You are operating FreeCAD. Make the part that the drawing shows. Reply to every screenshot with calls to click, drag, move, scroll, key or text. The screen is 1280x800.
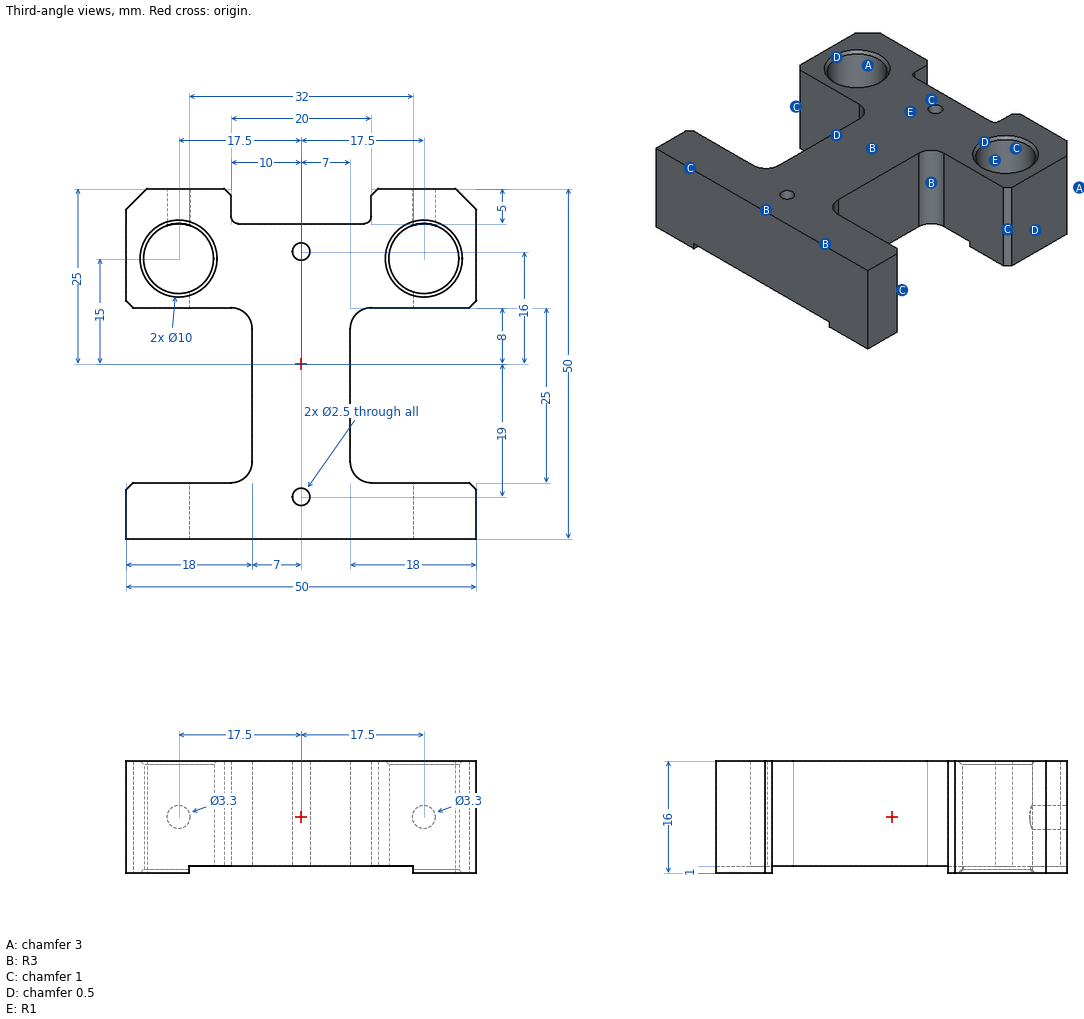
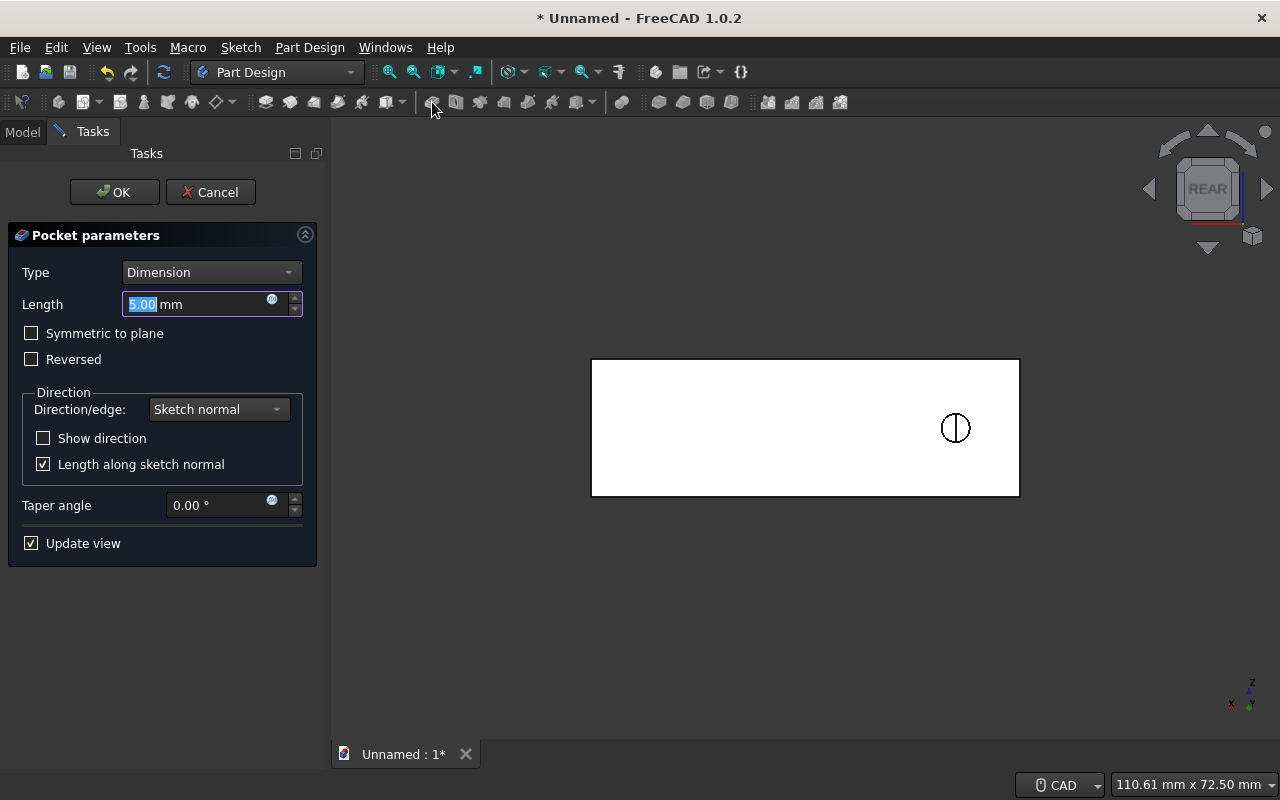
click(212, 272)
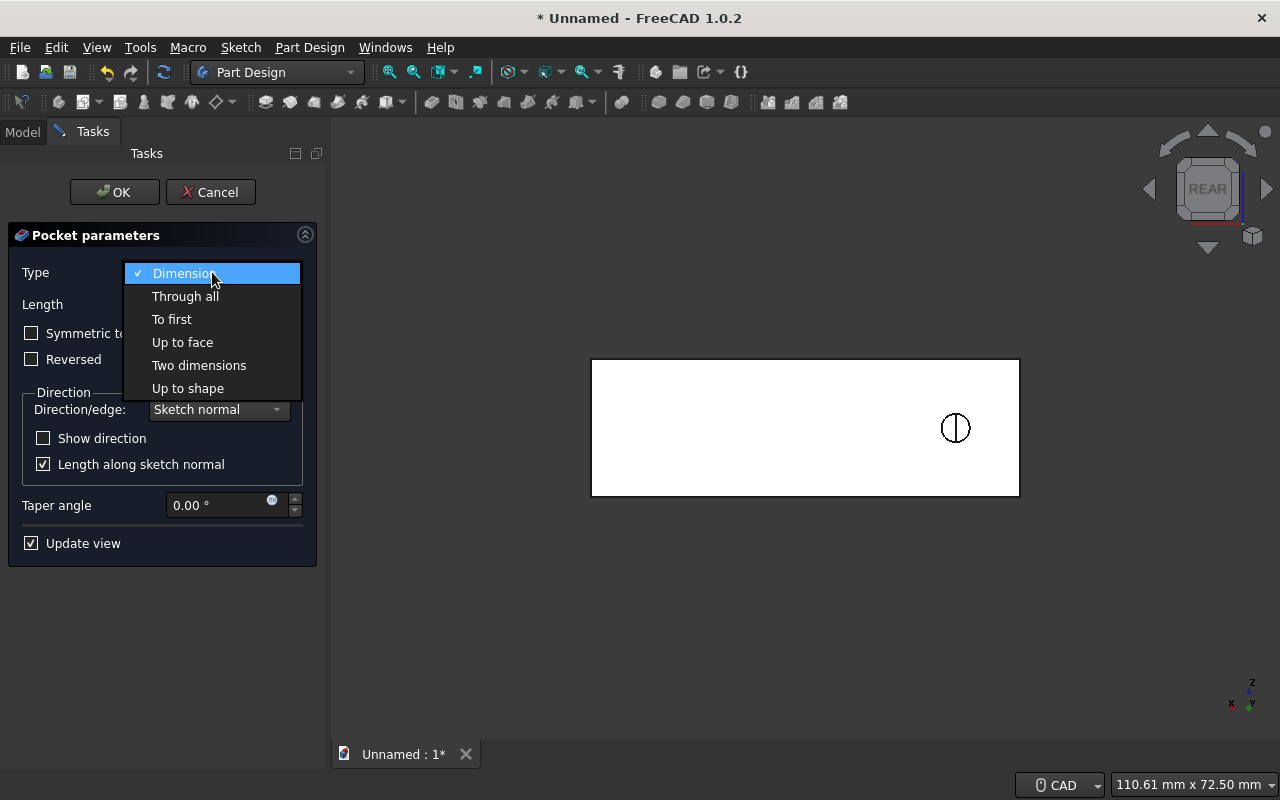
click(212, 320)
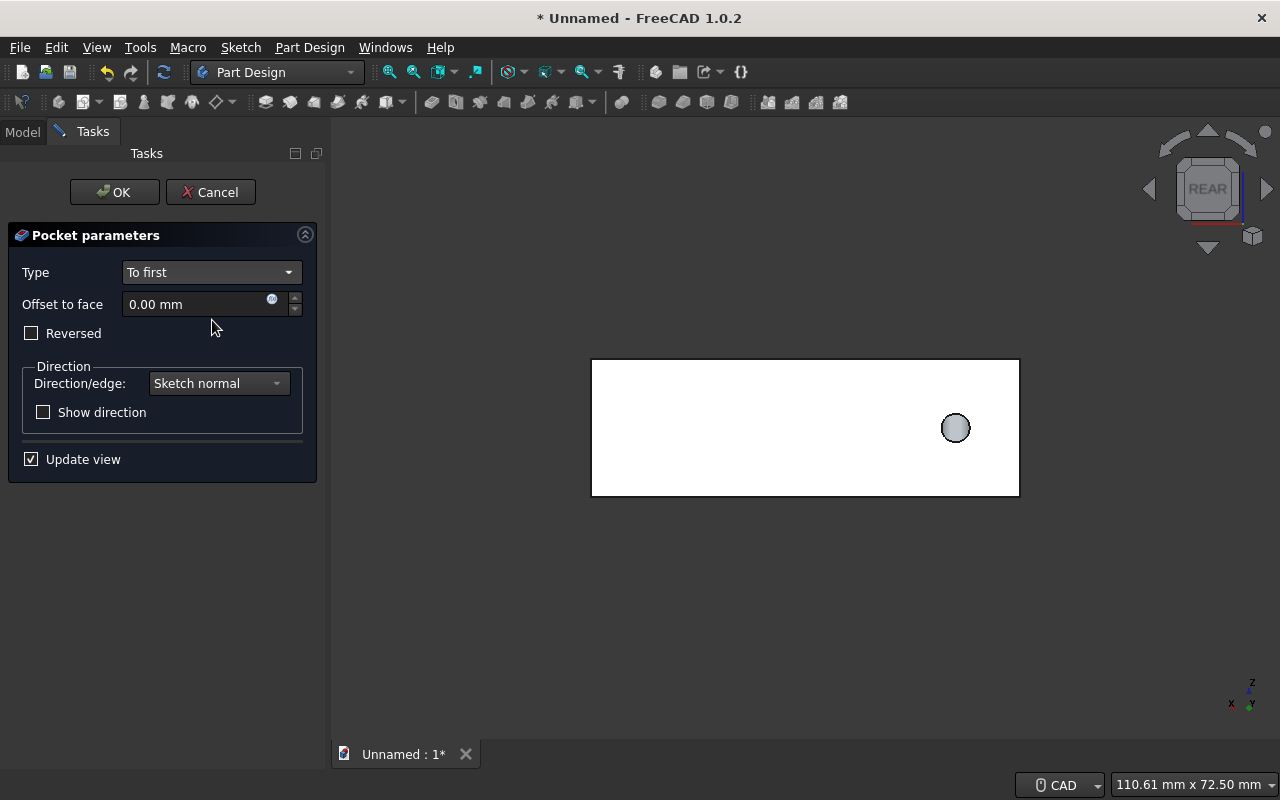
click(115, 192)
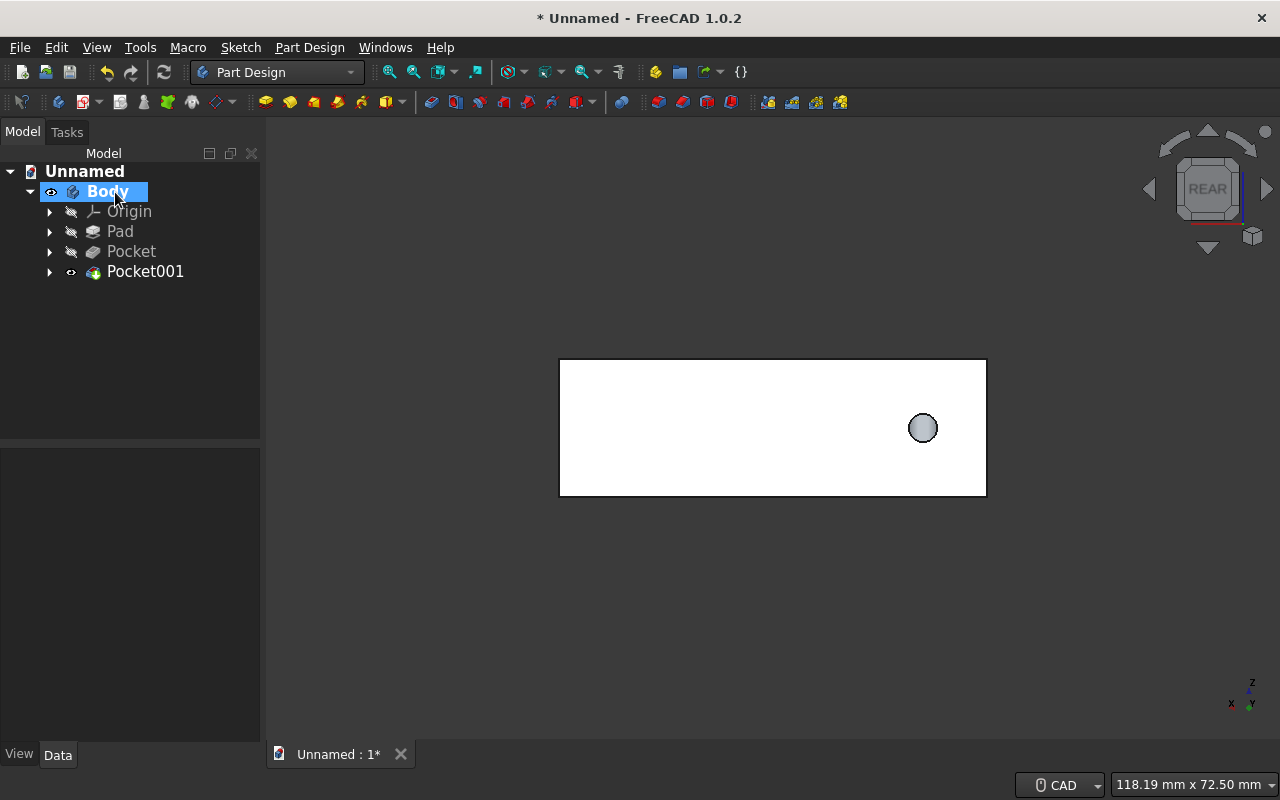
key(v)
key(f)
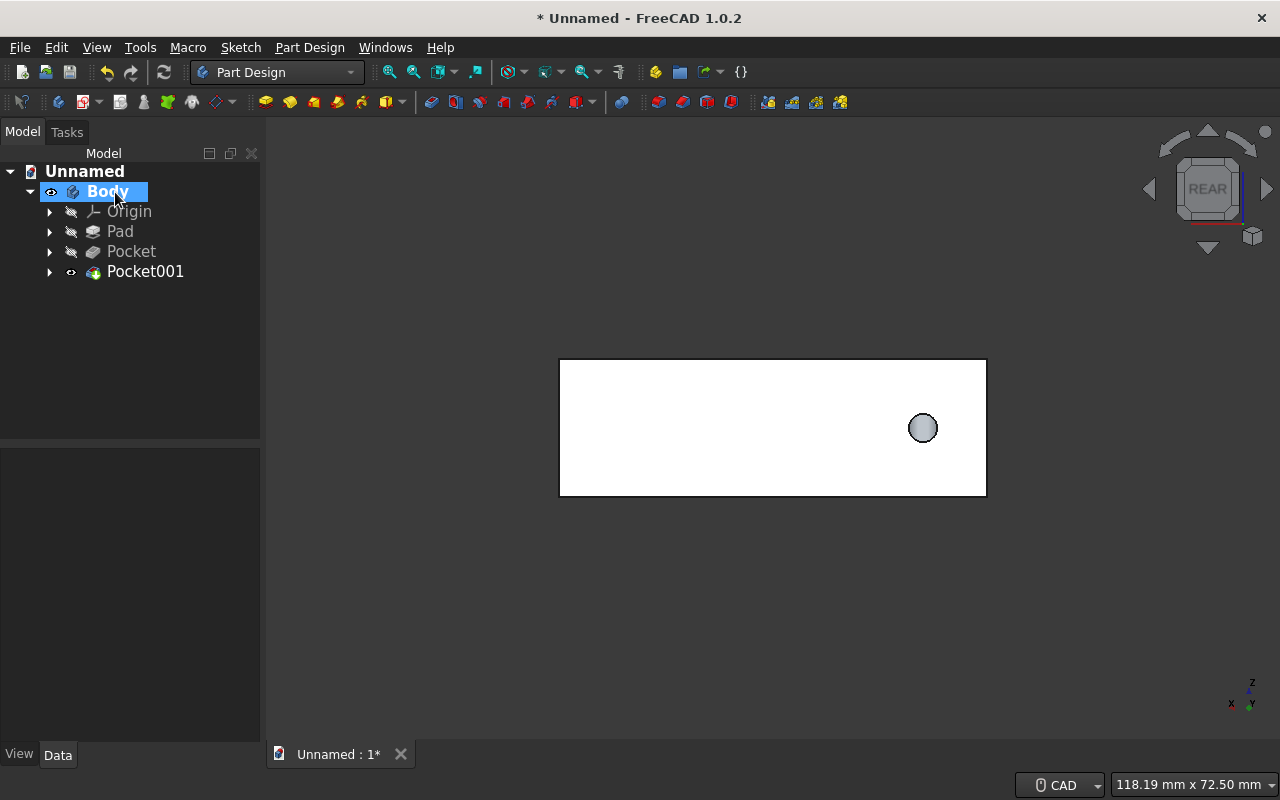
click(650, 427)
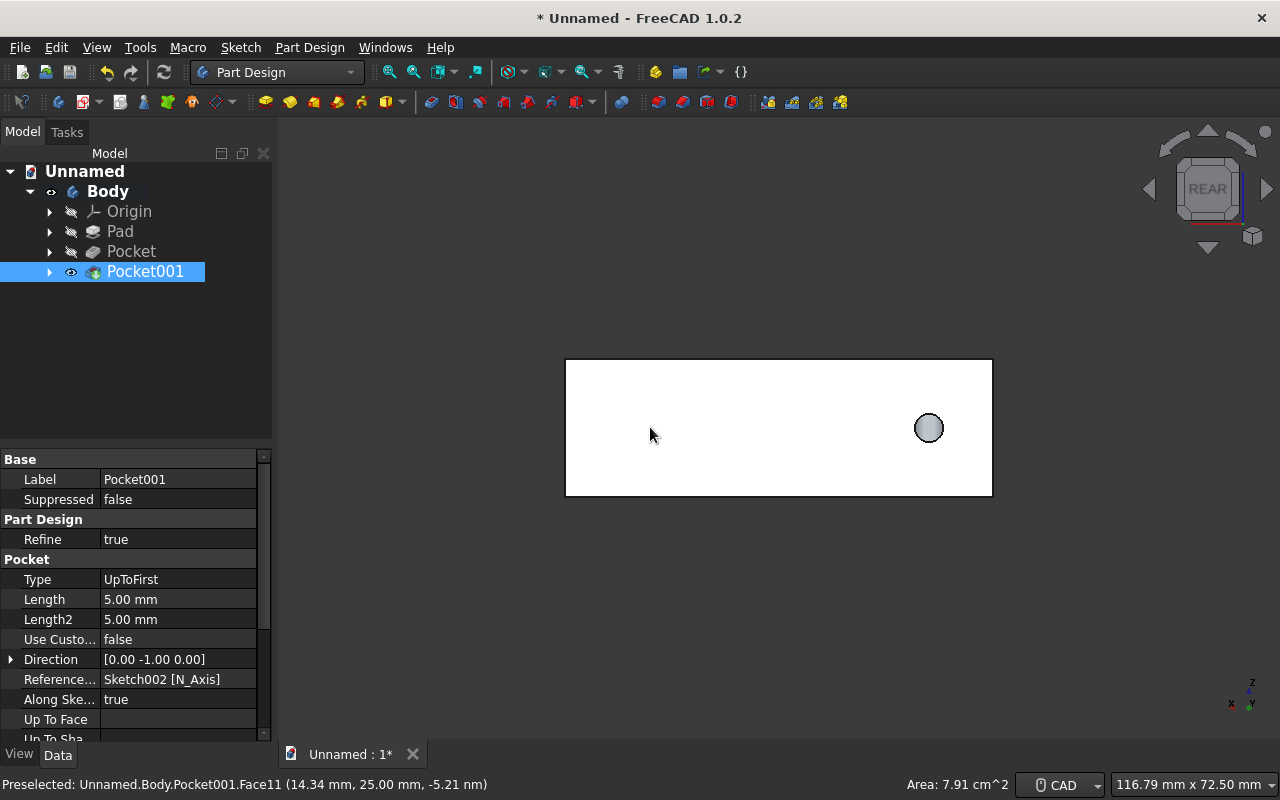
click(84, 102)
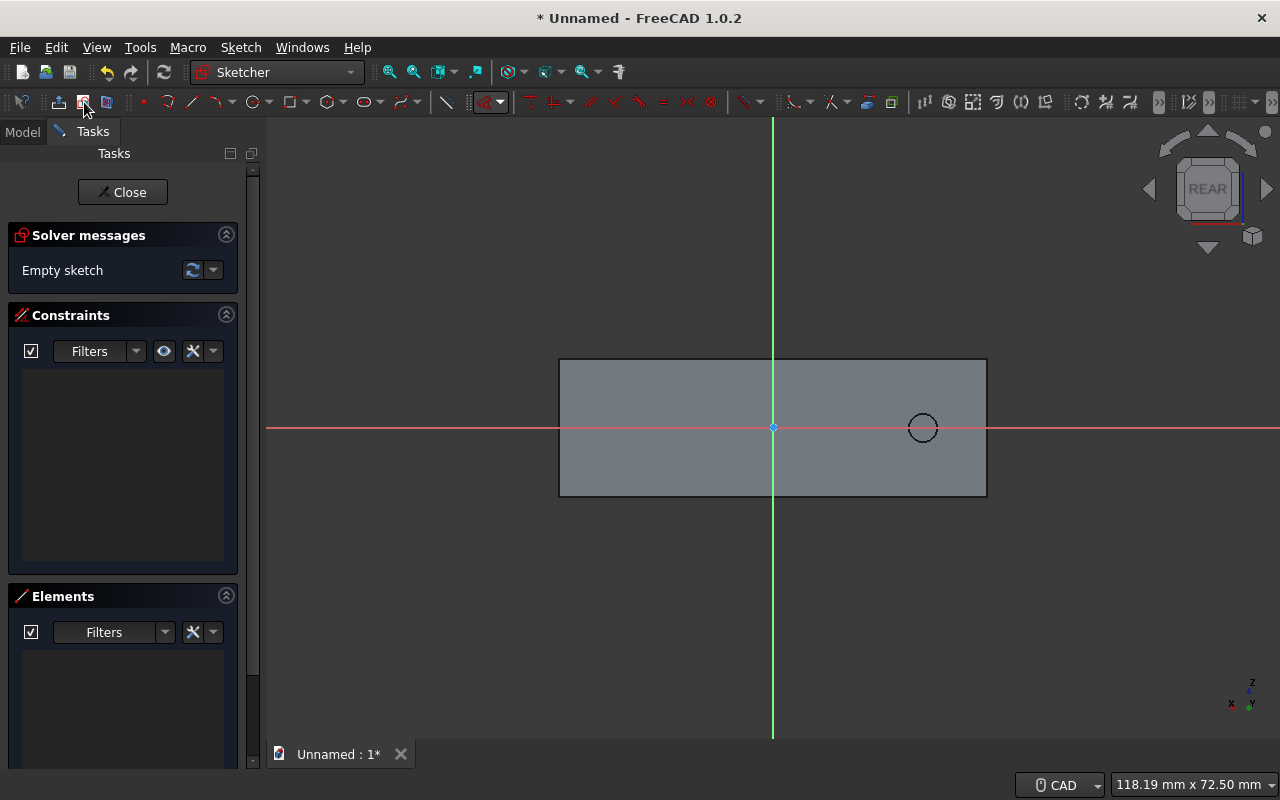
scroll(616, 428, up, 13)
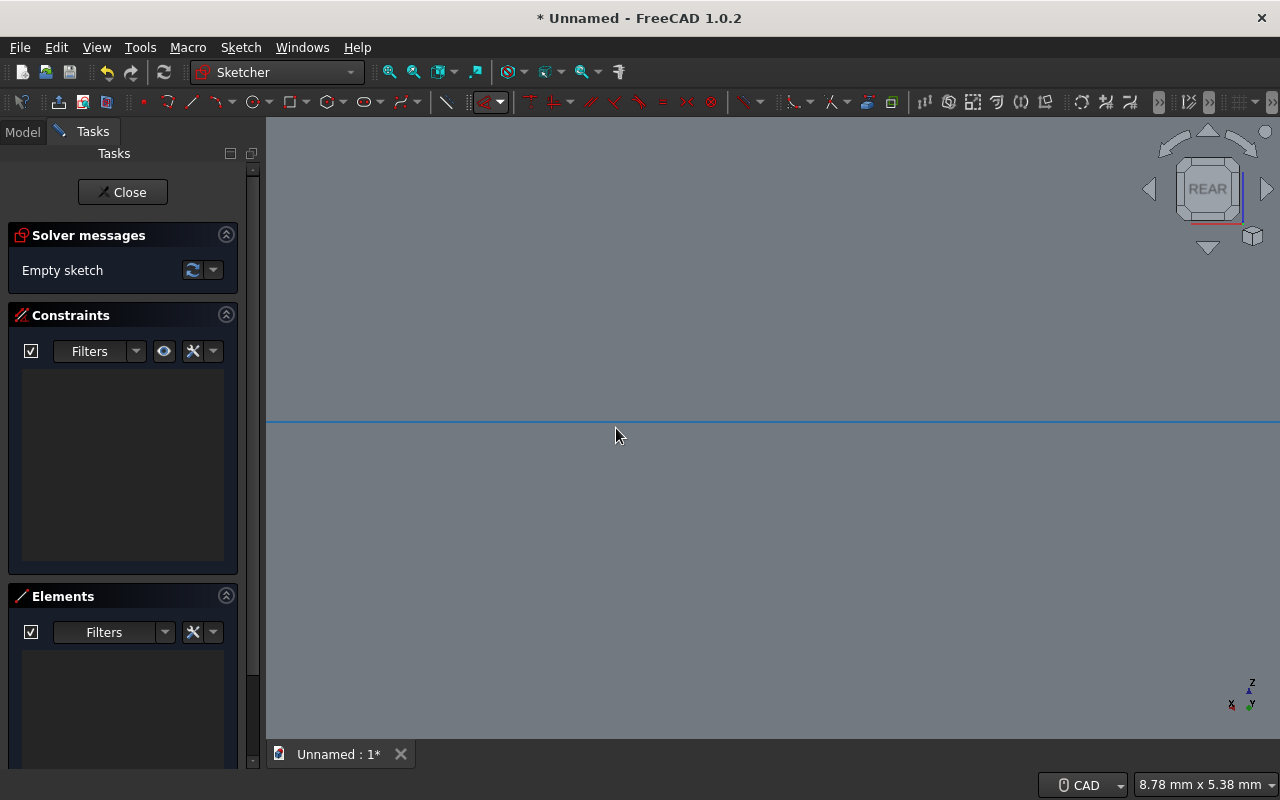
key(g)
key(c)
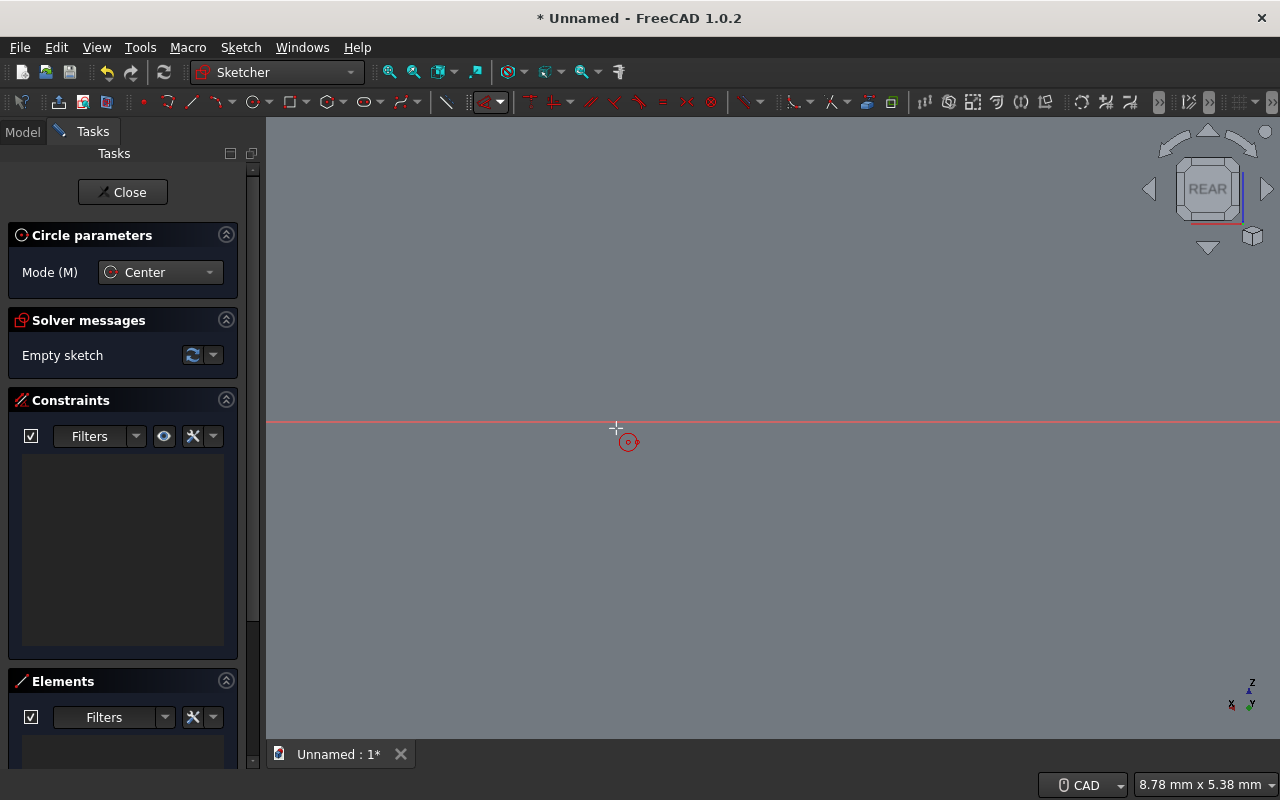
click(704, 422)
move(839, 287)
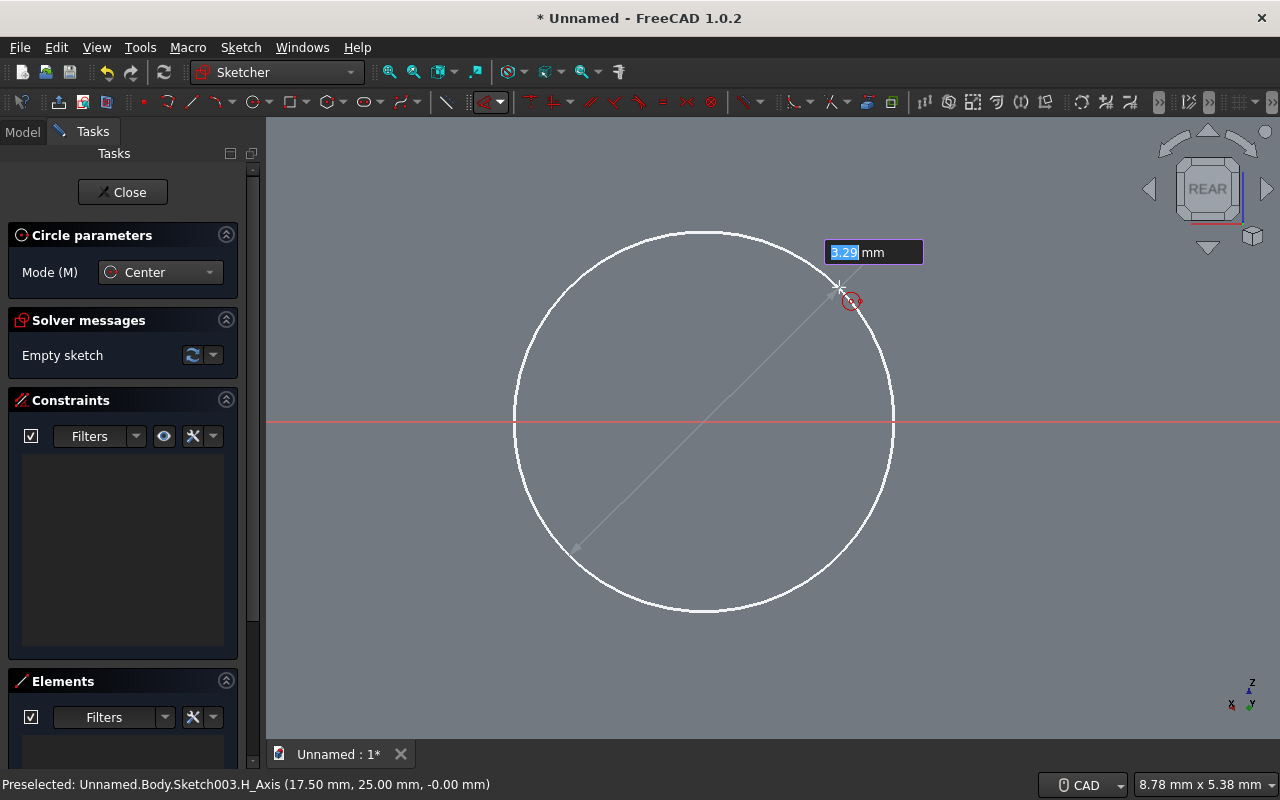
text(3.3)
key(Return)
key(Escape)